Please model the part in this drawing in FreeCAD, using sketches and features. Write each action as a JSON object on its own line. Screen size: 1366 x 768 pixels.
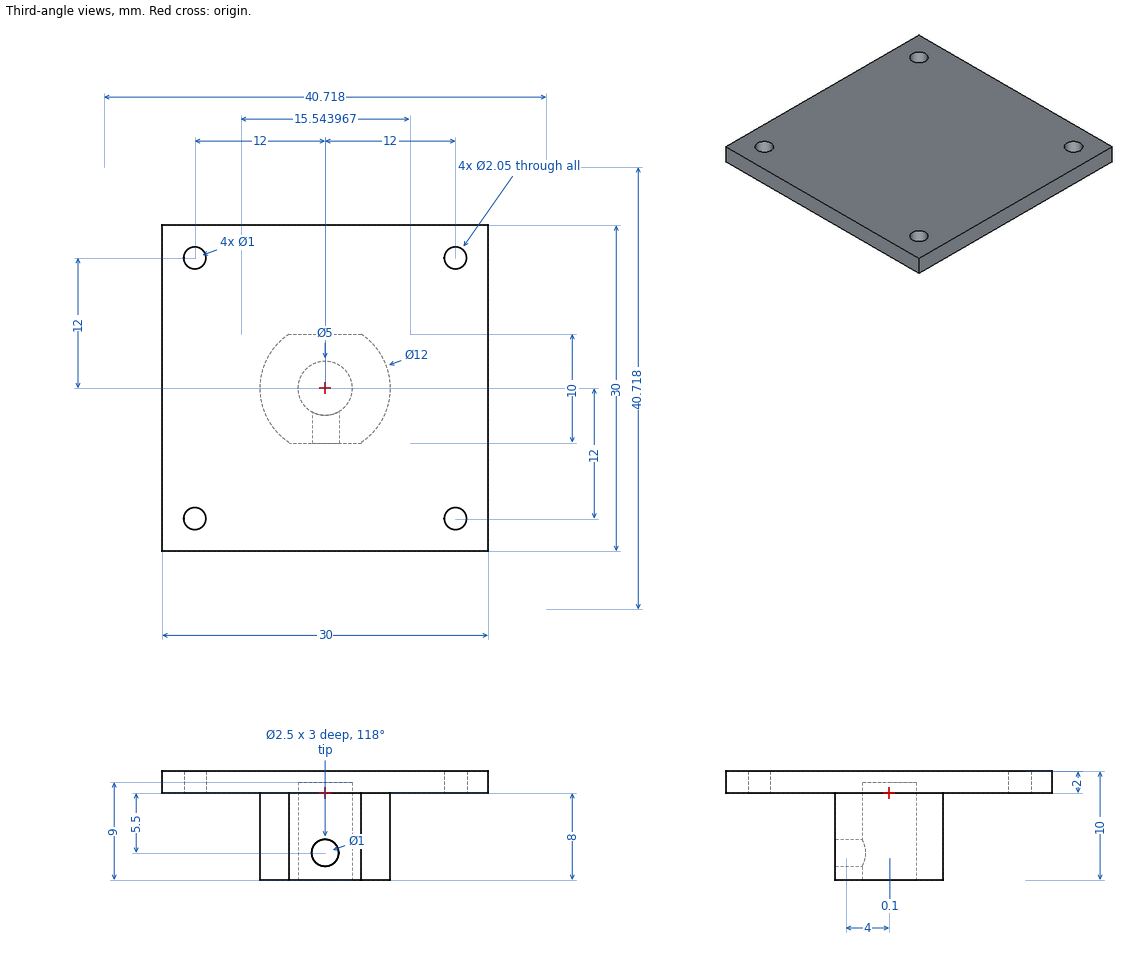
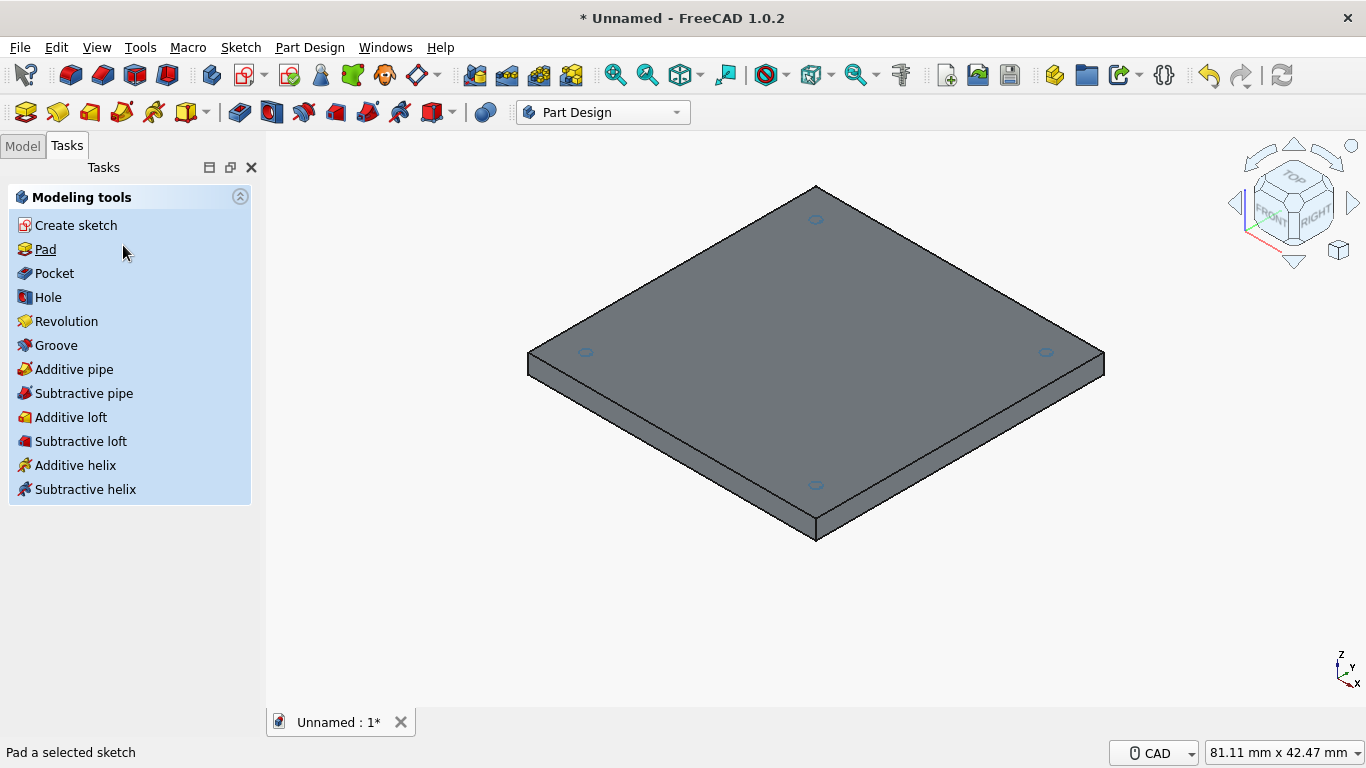
{"action": "left_click", "coordinate": [240, 112]}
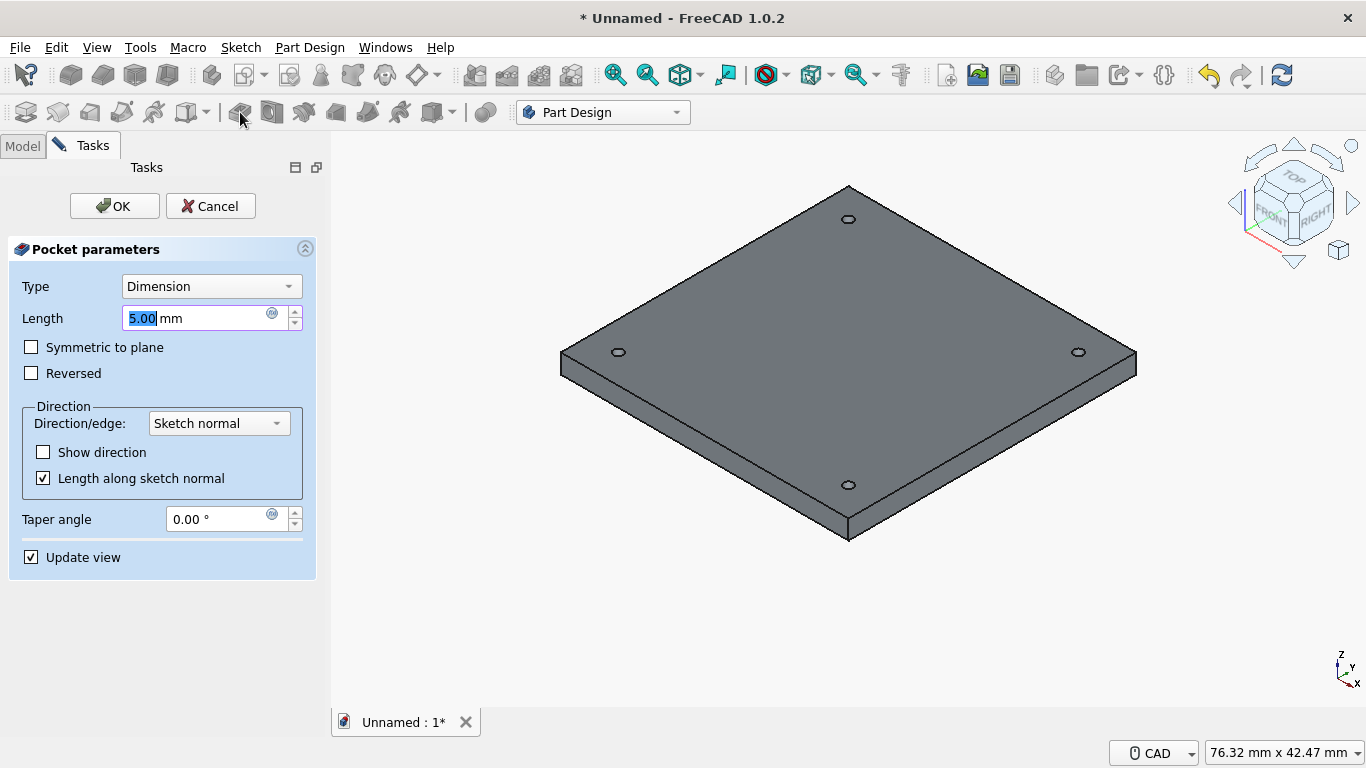
{"action": "type", "text": "10"}
{"action": "key", "text": "Tab"}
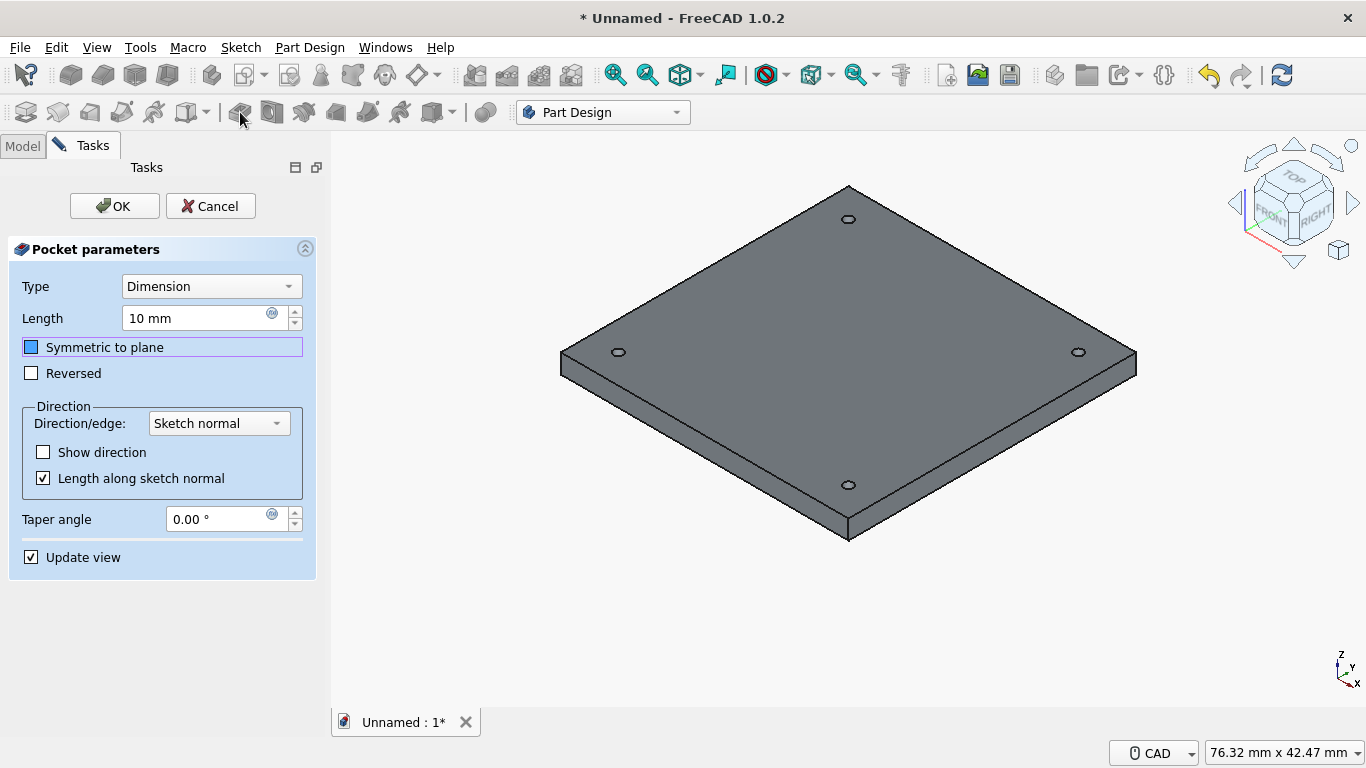
{"action": "left_click", "coordinate": [115, 206]}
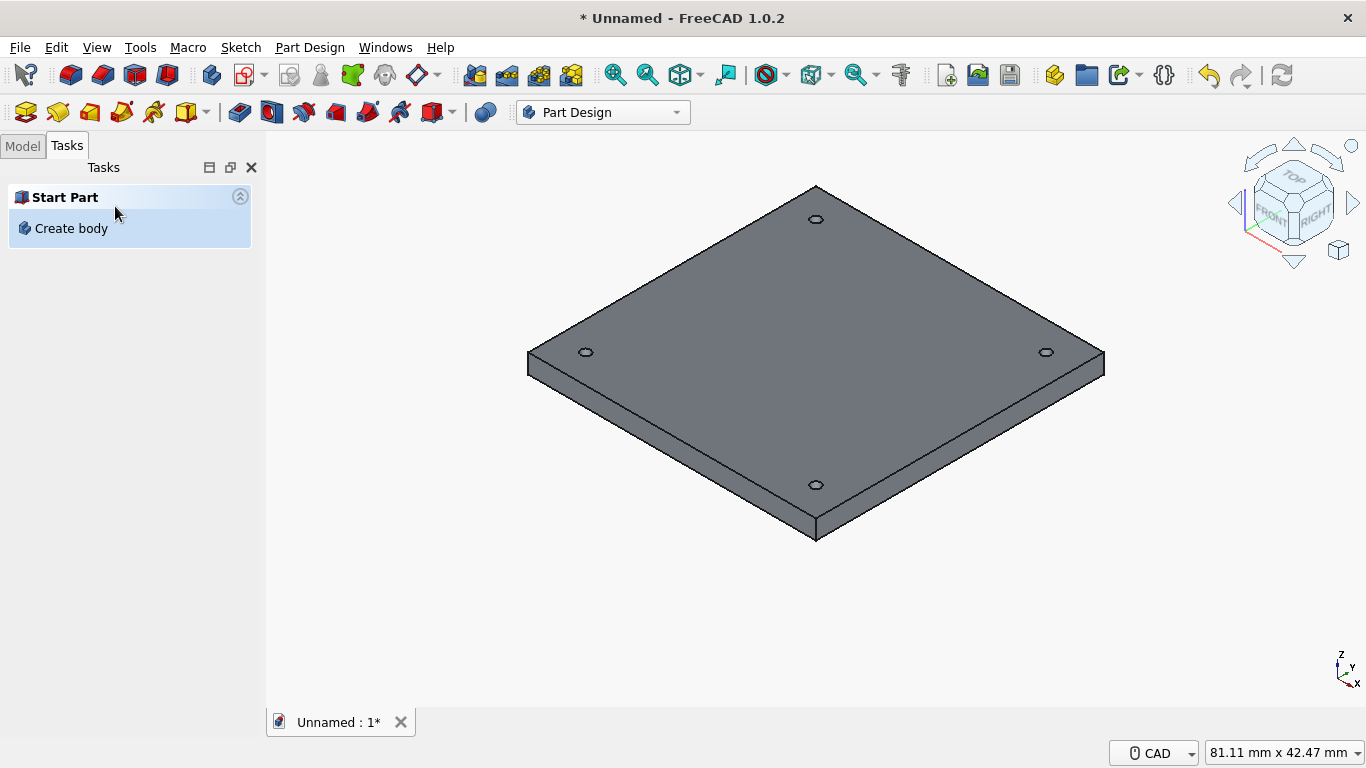
{"action": "key", "text": "5"}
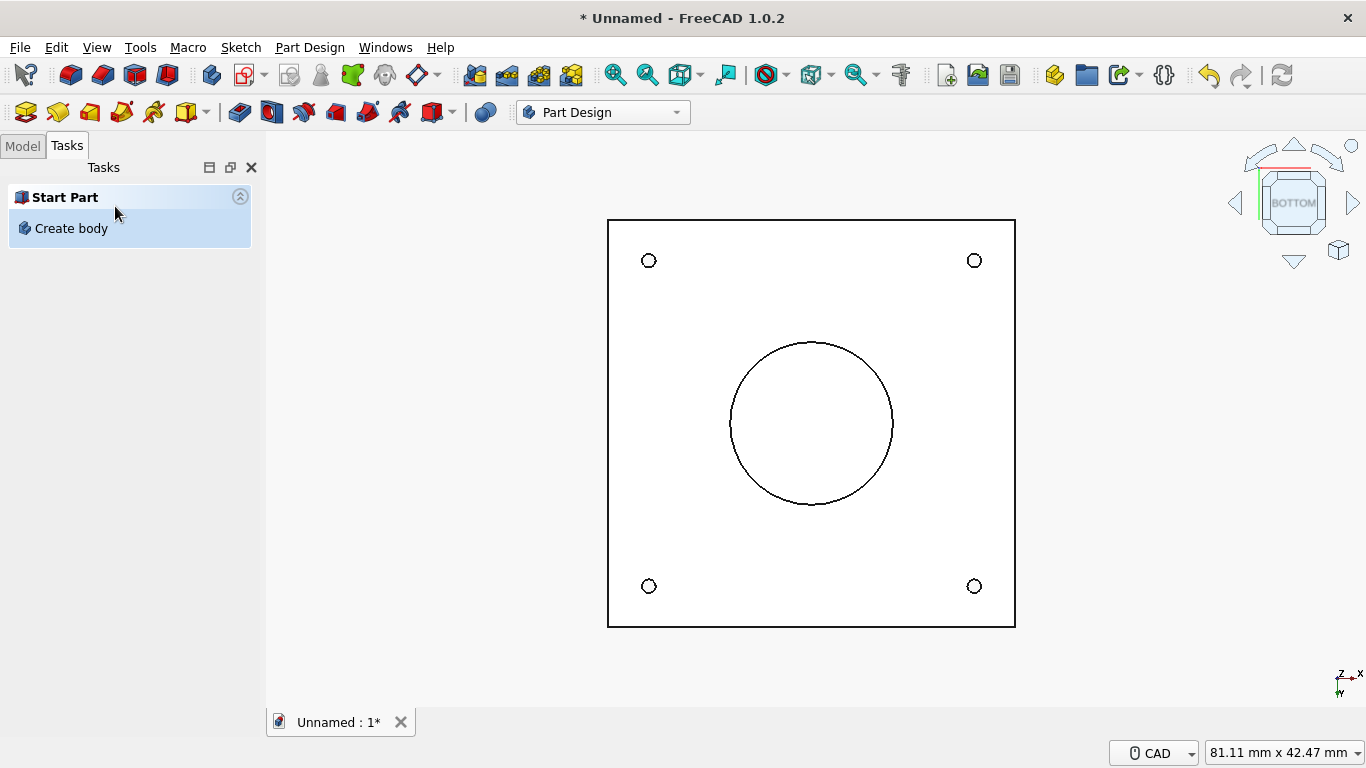
{"action": "left_click", "coordinate": [812, 422]}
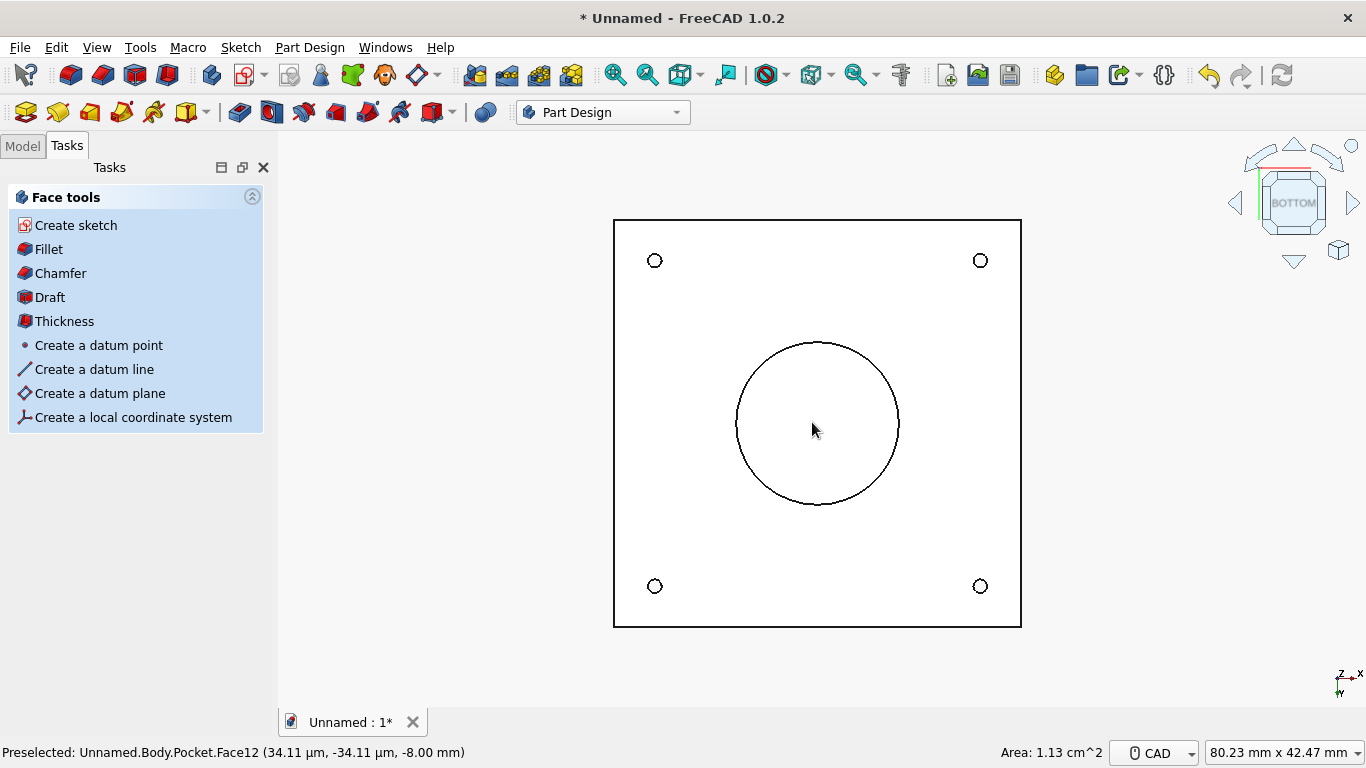
{"action": "left_click", "coordinate": [244, 76]}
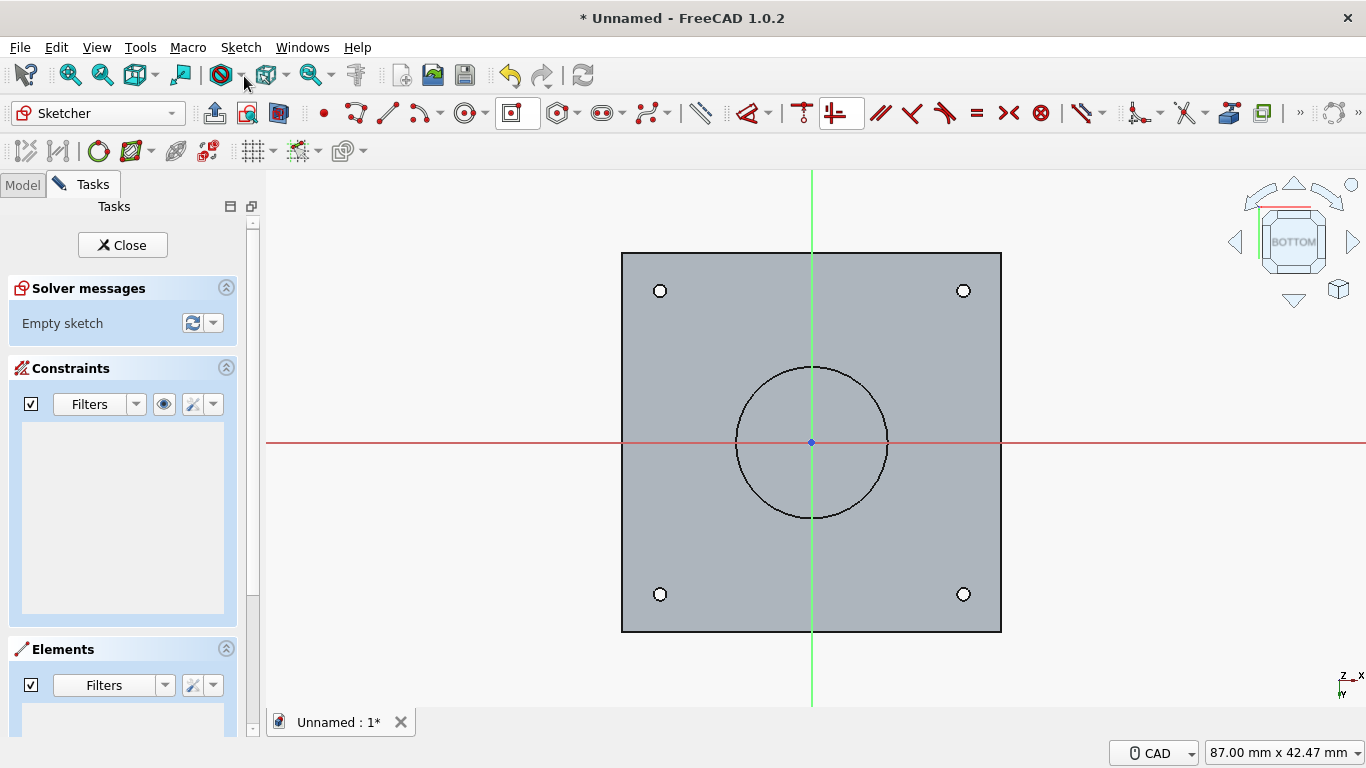
{"action": "scroll", "coordinate": [828, 444], "scroll_direction": "up", "scroll_amount": 8}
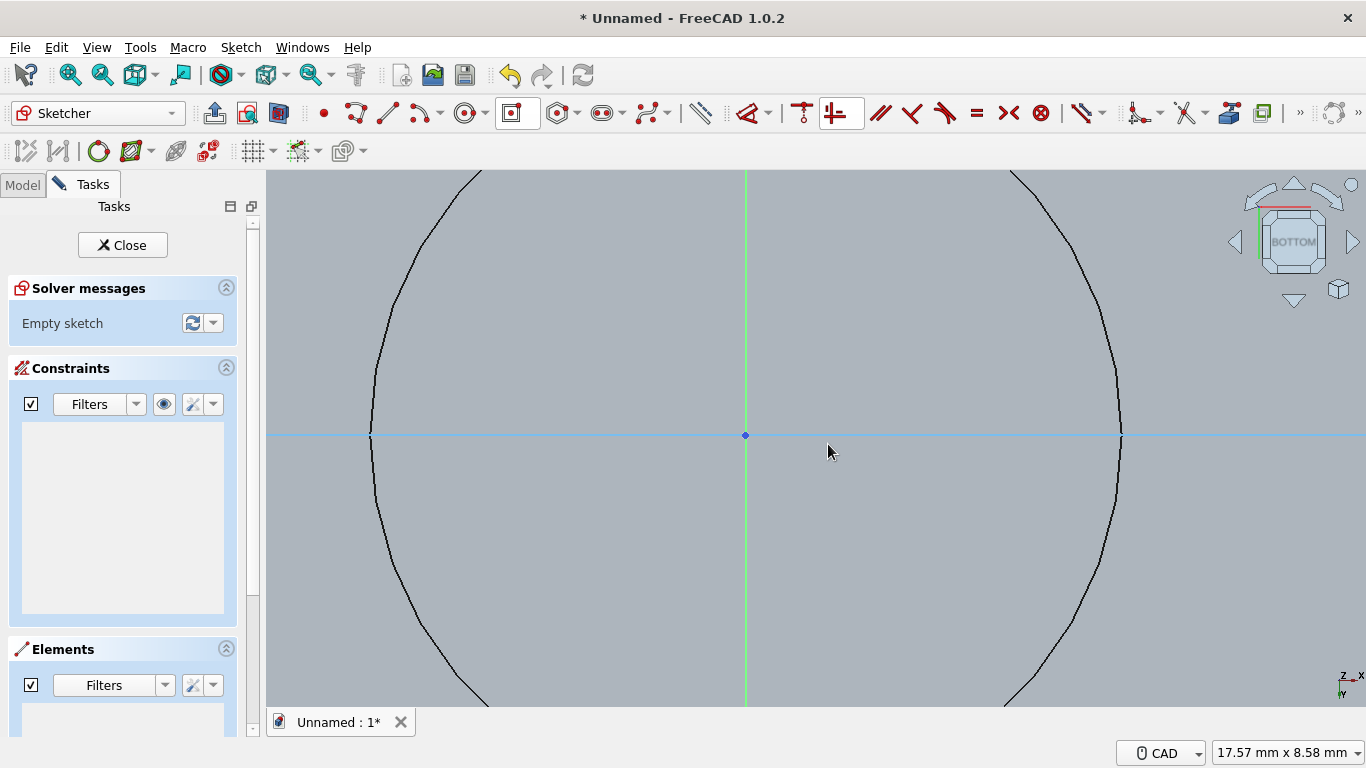
{"action": "key", "text": "g c"}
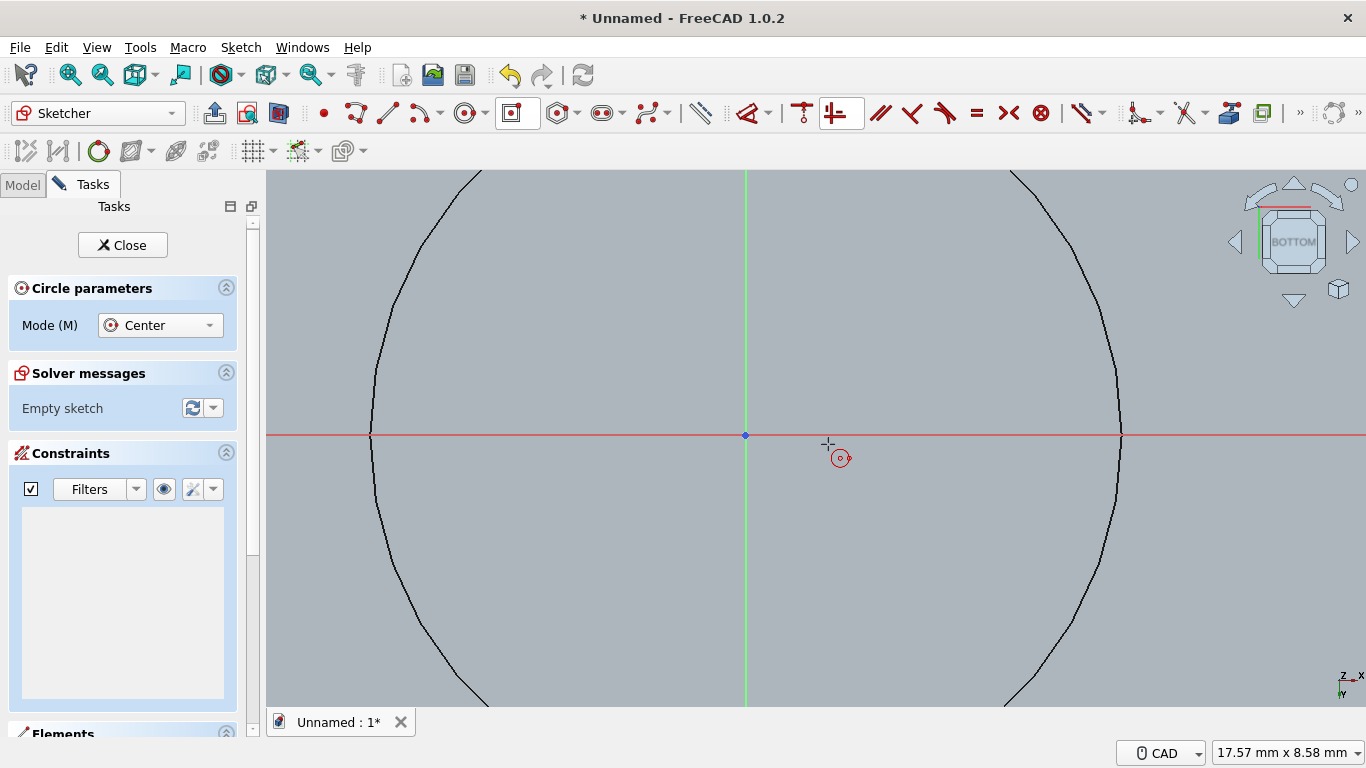
{"action": "left_click", "coordinate": [746, 435]}
{"action": "left_click", "coordinate": [857, 325]}
{"action": "key", "text": "Escape"}